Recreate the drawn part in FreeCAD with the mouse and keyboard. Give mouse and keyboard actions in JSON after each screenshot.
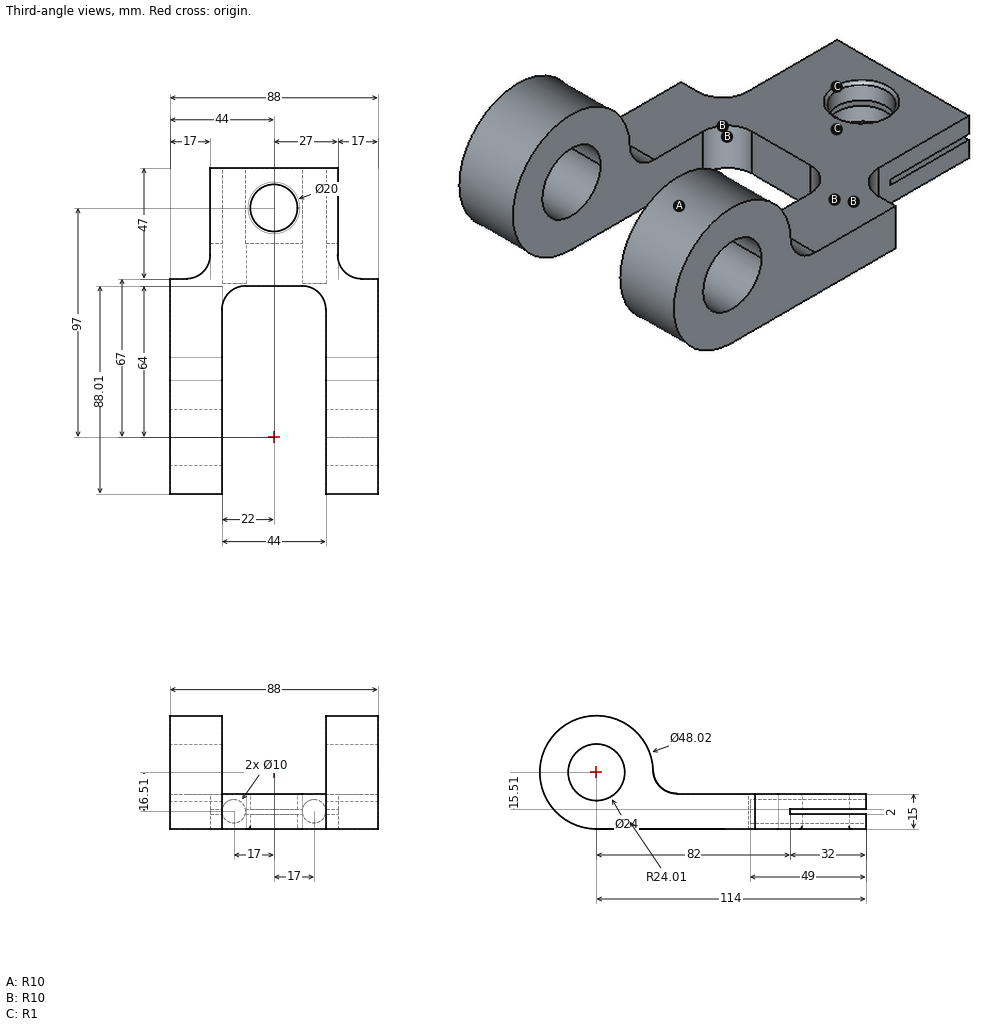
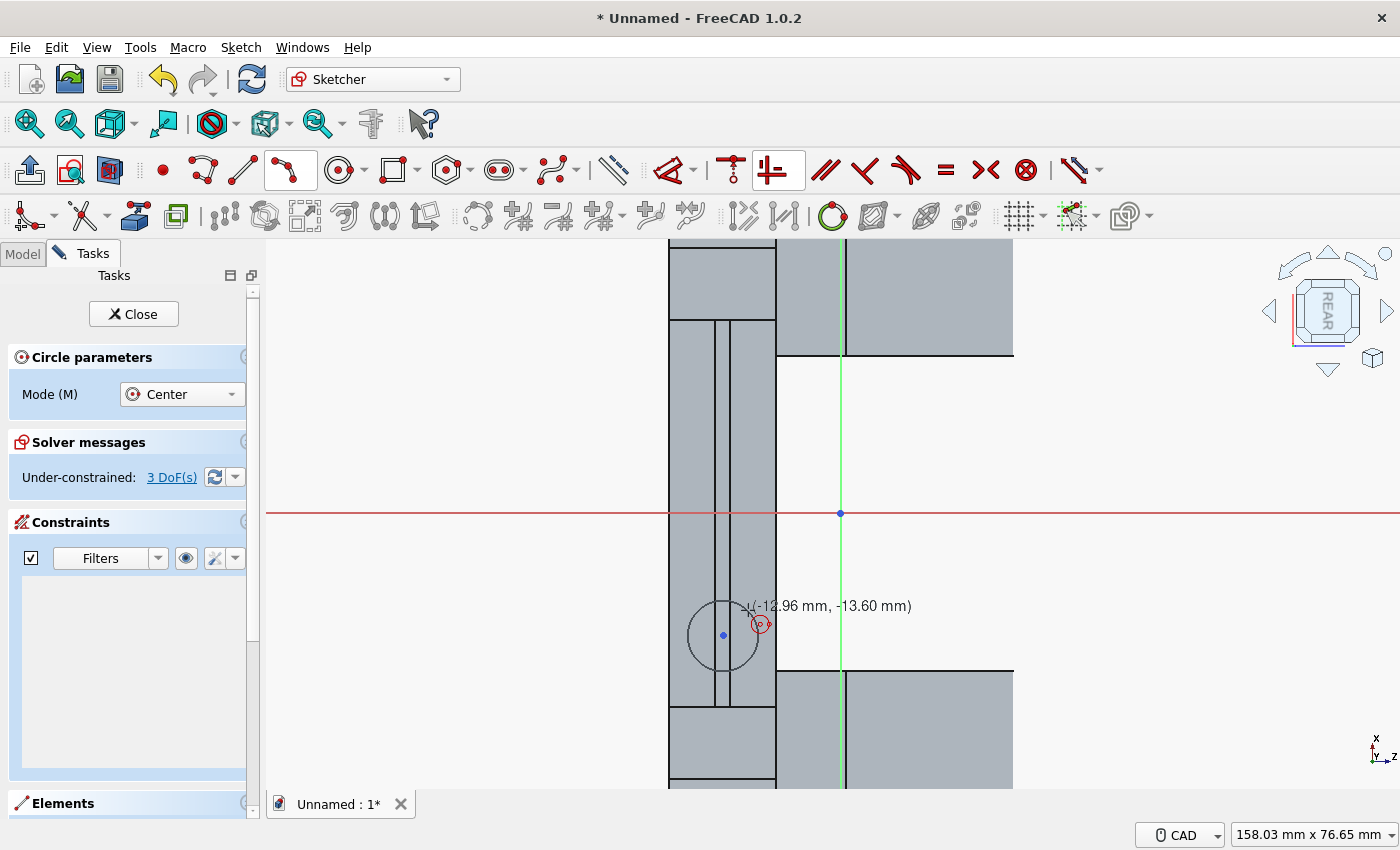
{"action": "left_click", "coordinate": [723, 391]}
{"action": "left_click", "coordinate": [748, 366]}
{"action": "key", "text": "Escape"}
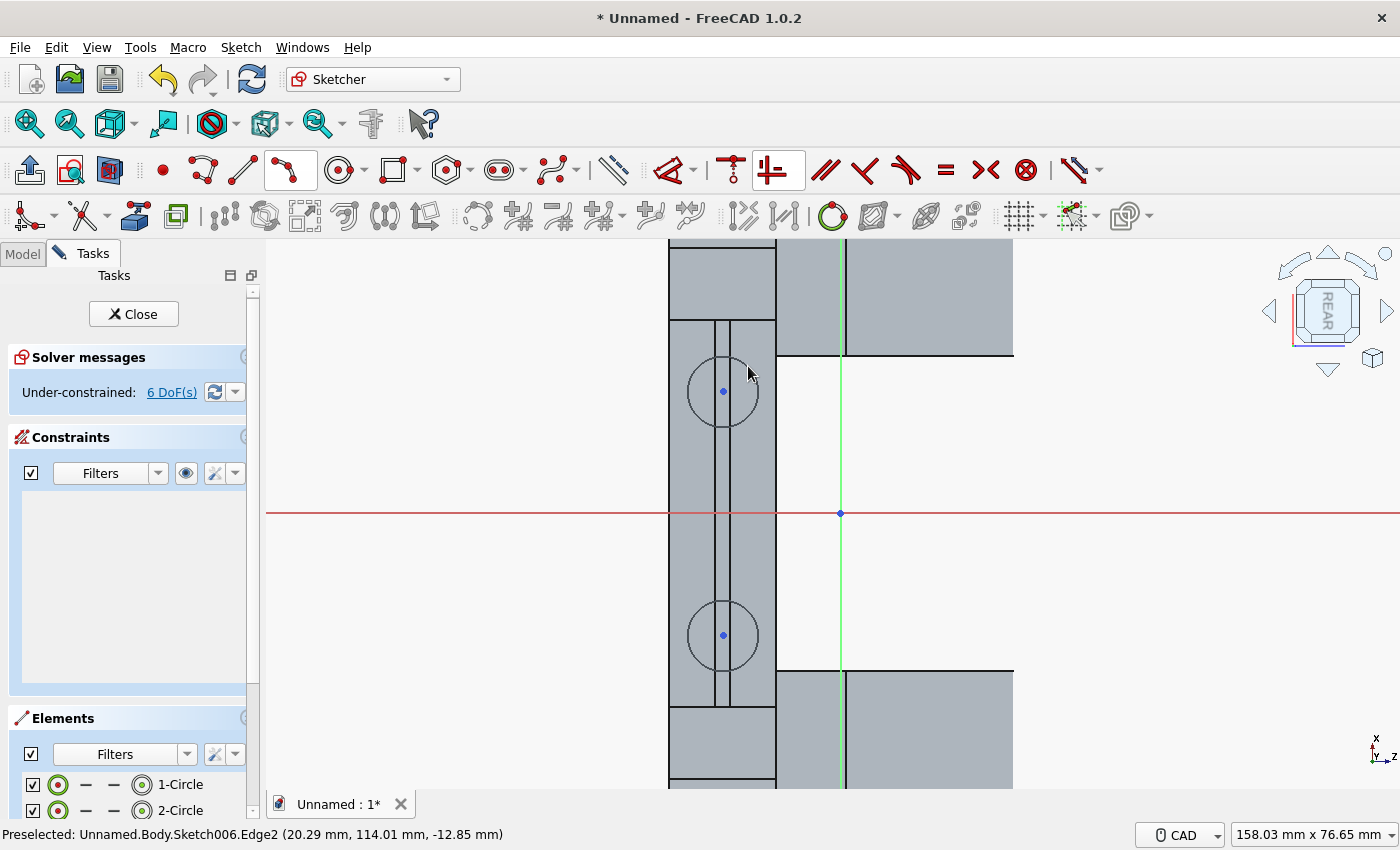
{"action": "left_click", "coordinate": [748, 611]}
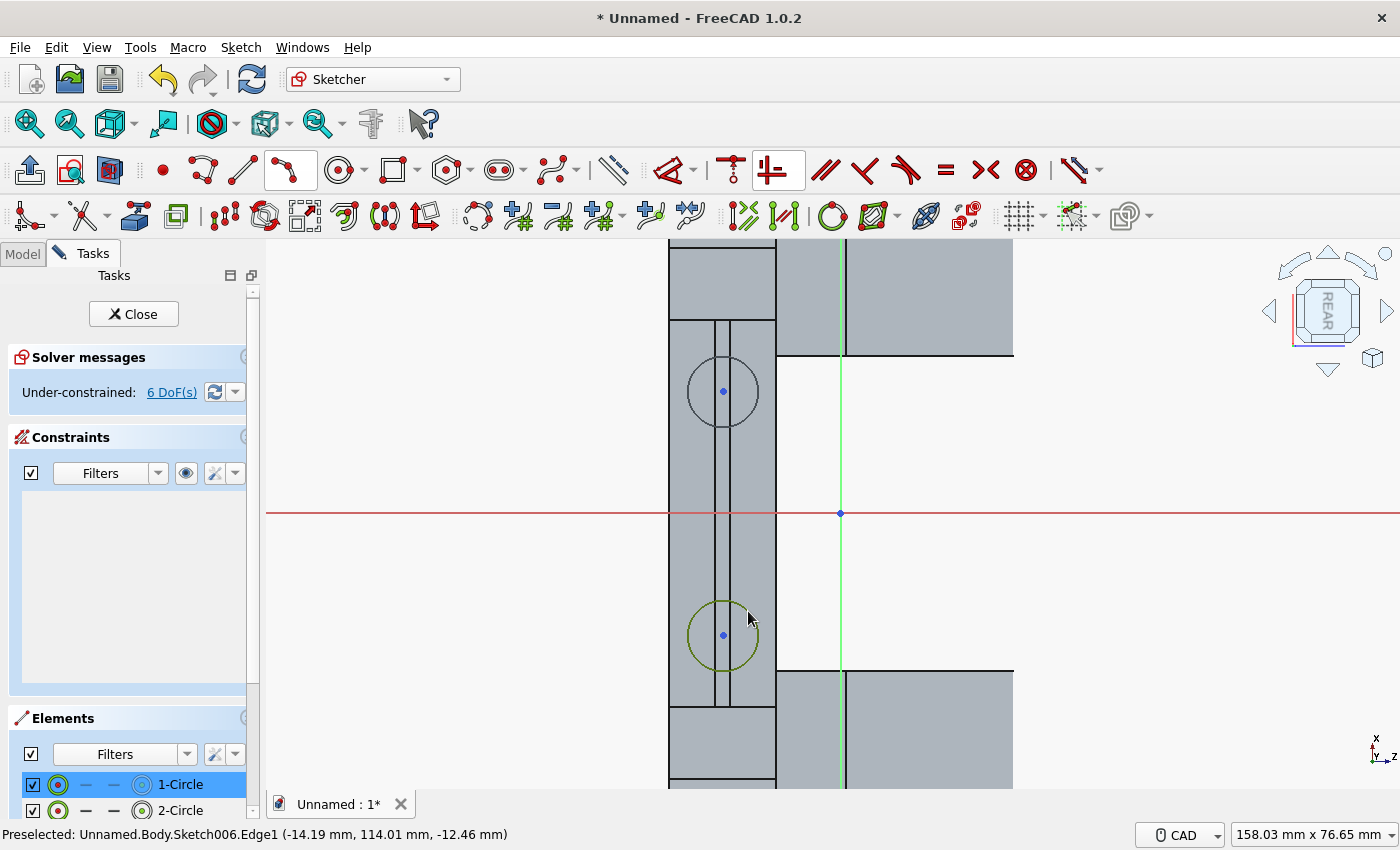
{"action": "left_click", "coordinate": [748, 367]}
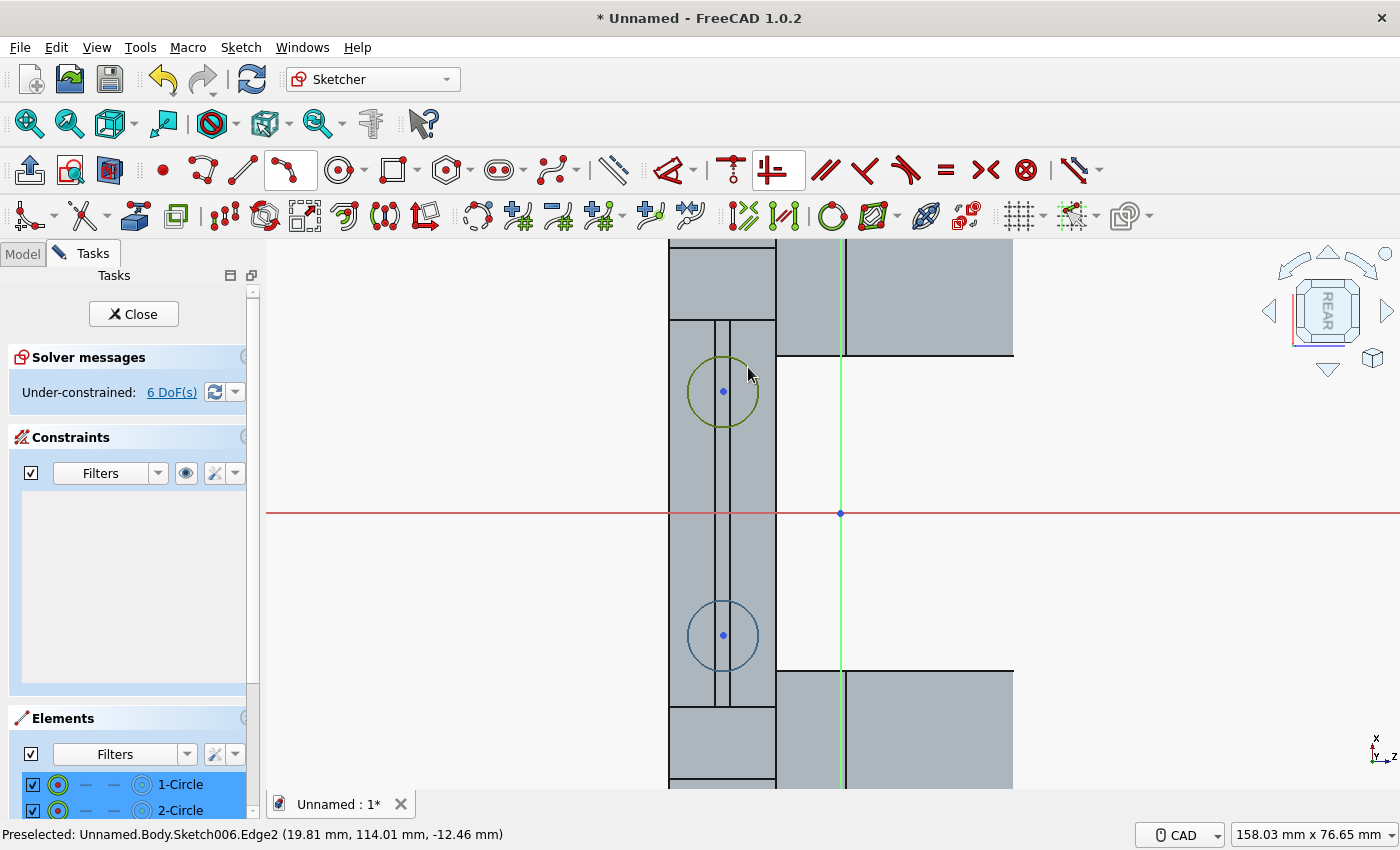
{"action": "left_click", "coordinate": [946, 170]}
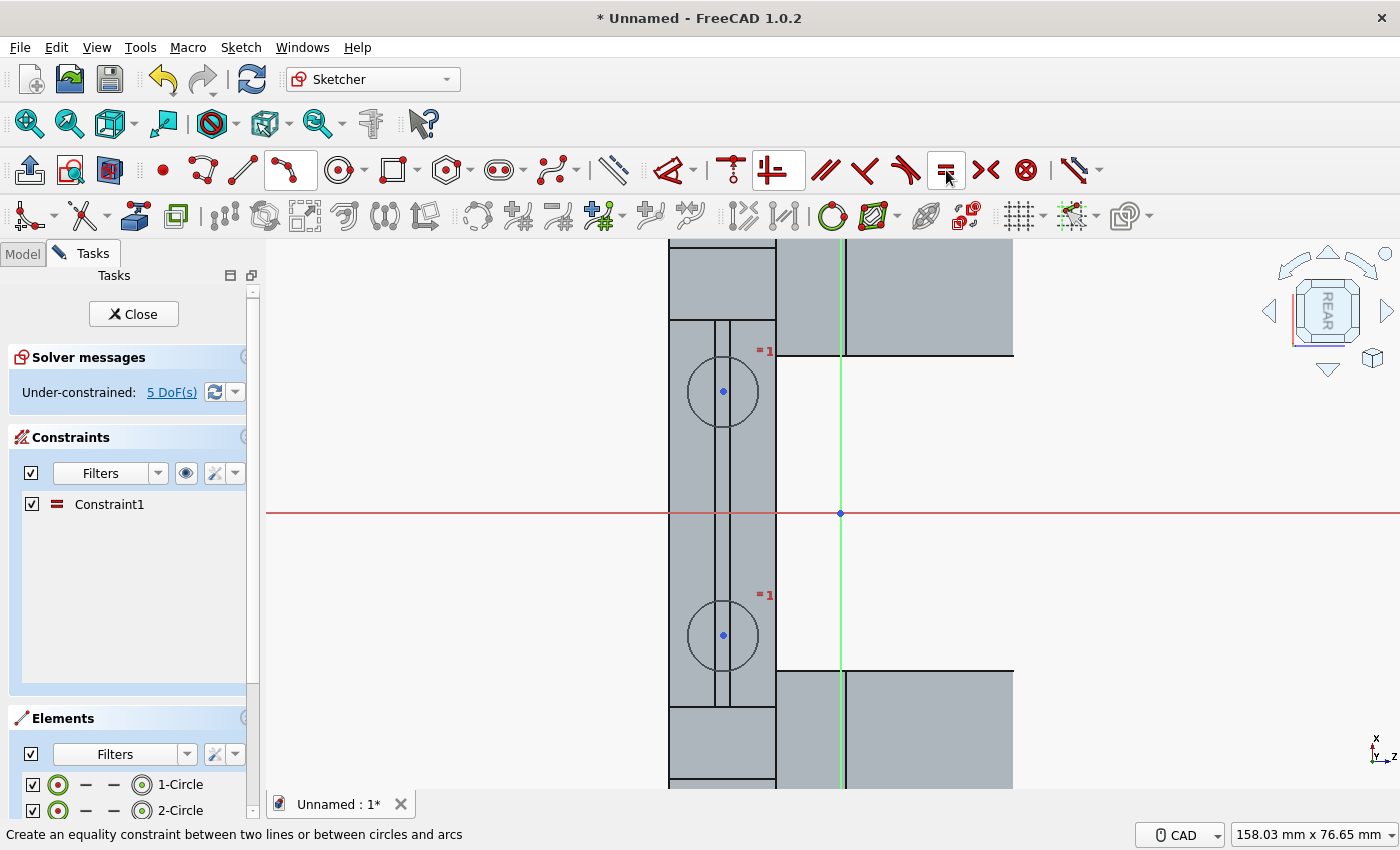
{"action": "left_click", "coordinate": [723, 636]}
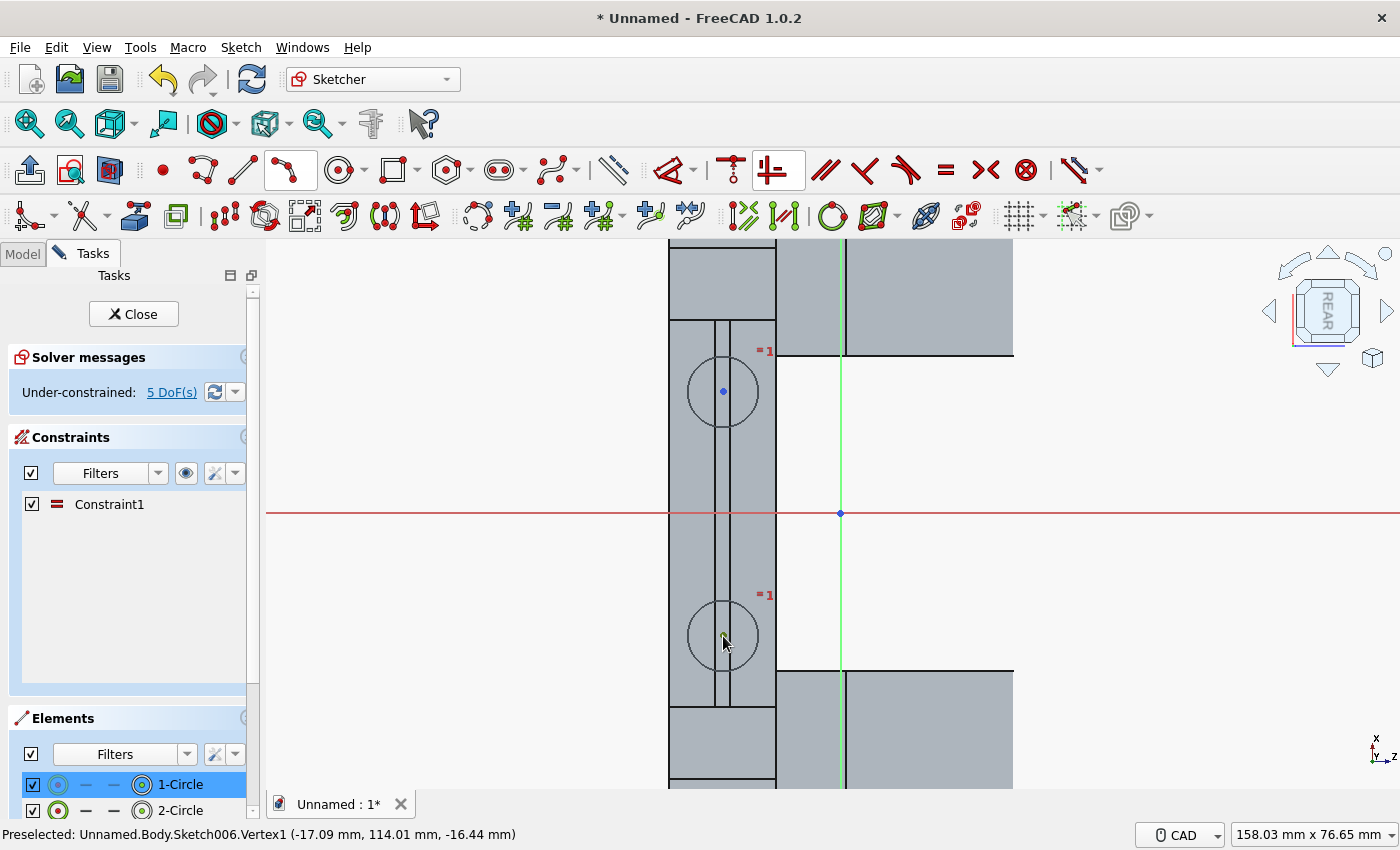
{"action": "left_click", "coordinate": [723, 392]}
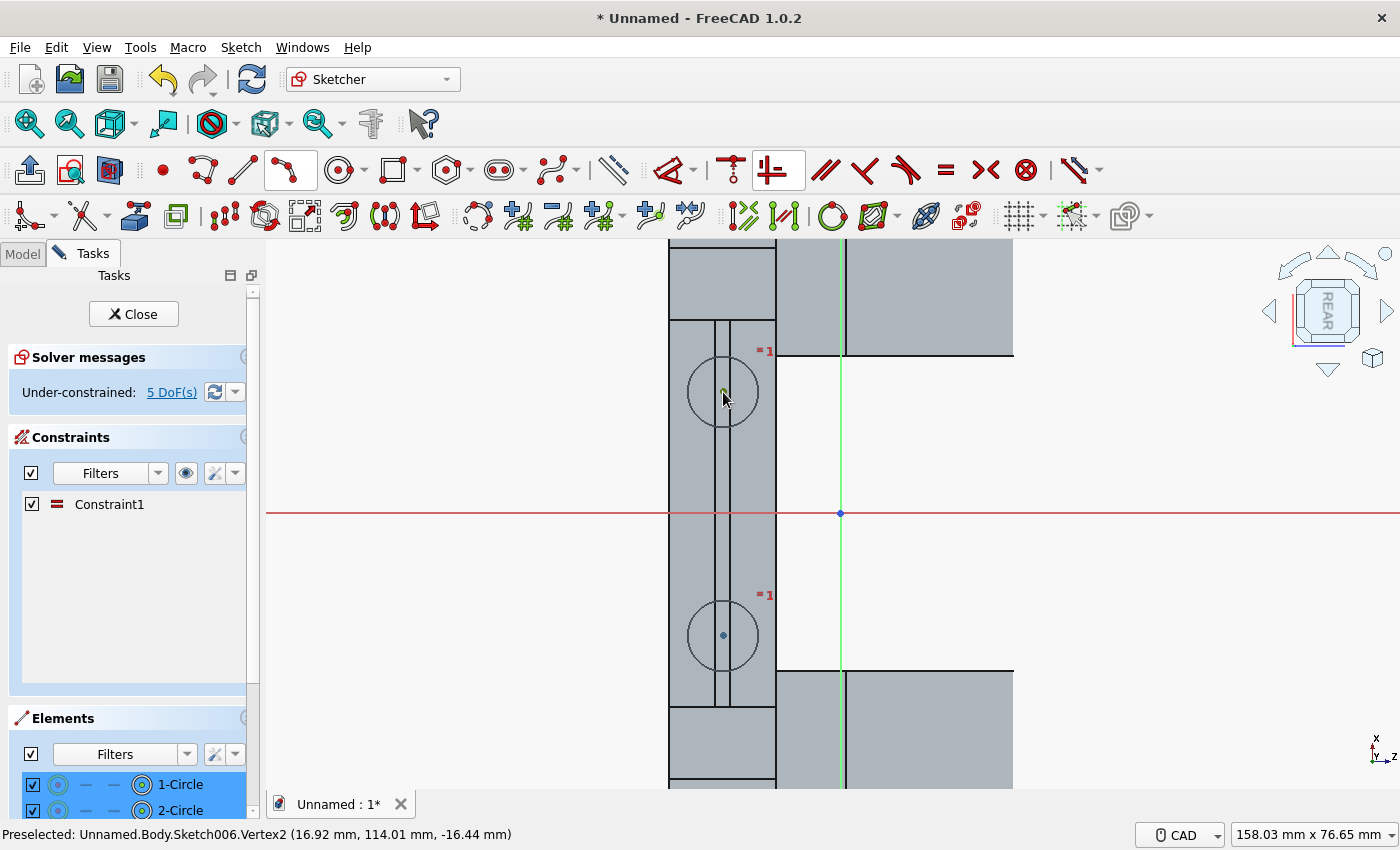
{"action": "key", "text": "v"}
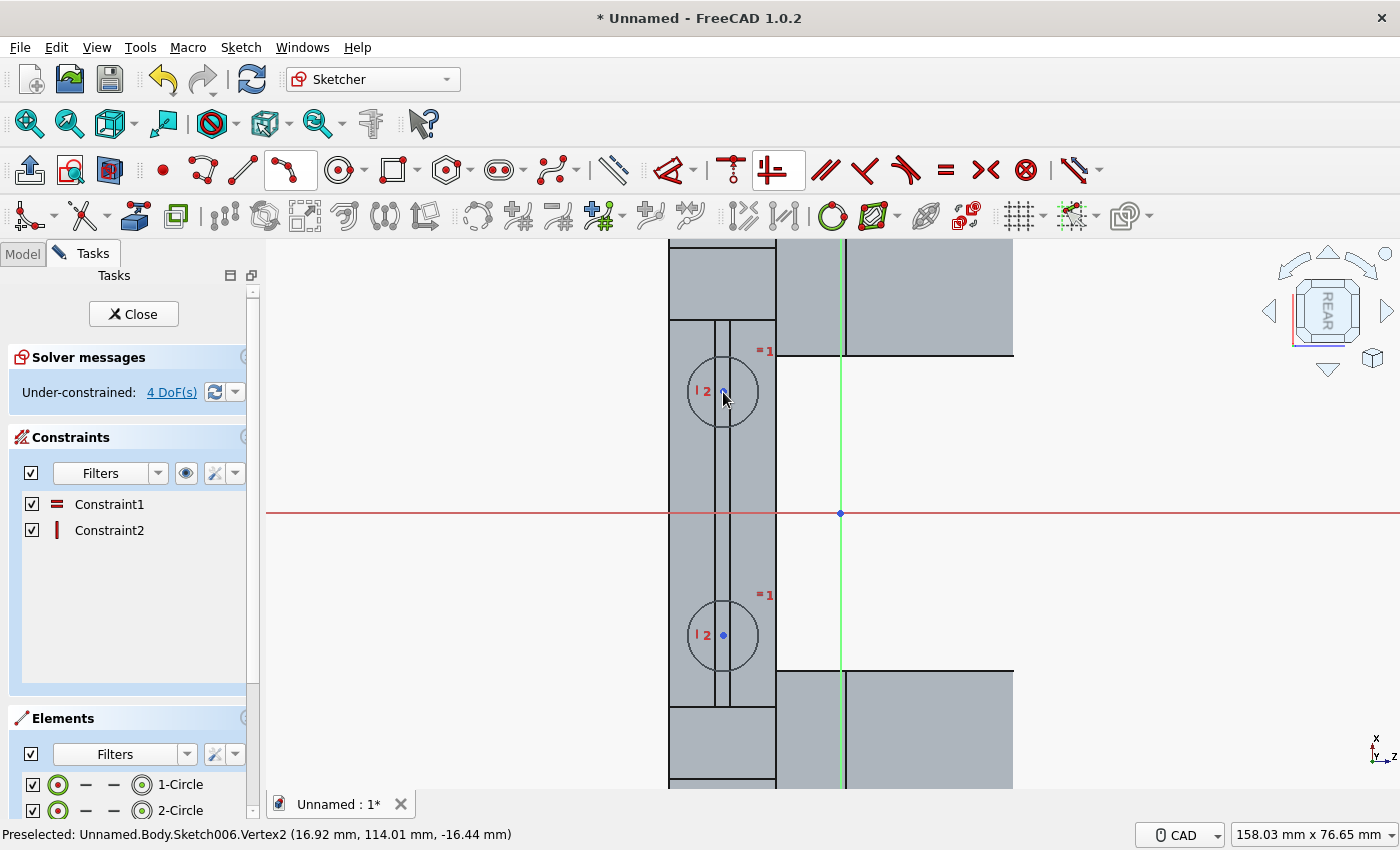
{"action": "left_click", "coordinate": [668, 170]}